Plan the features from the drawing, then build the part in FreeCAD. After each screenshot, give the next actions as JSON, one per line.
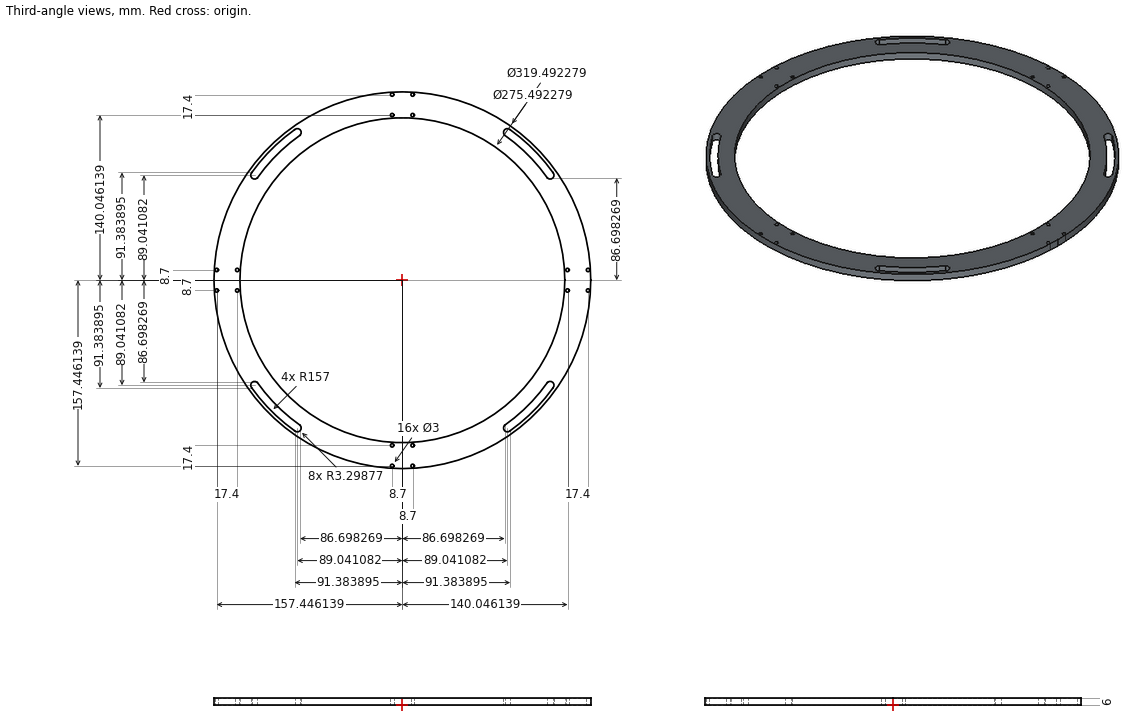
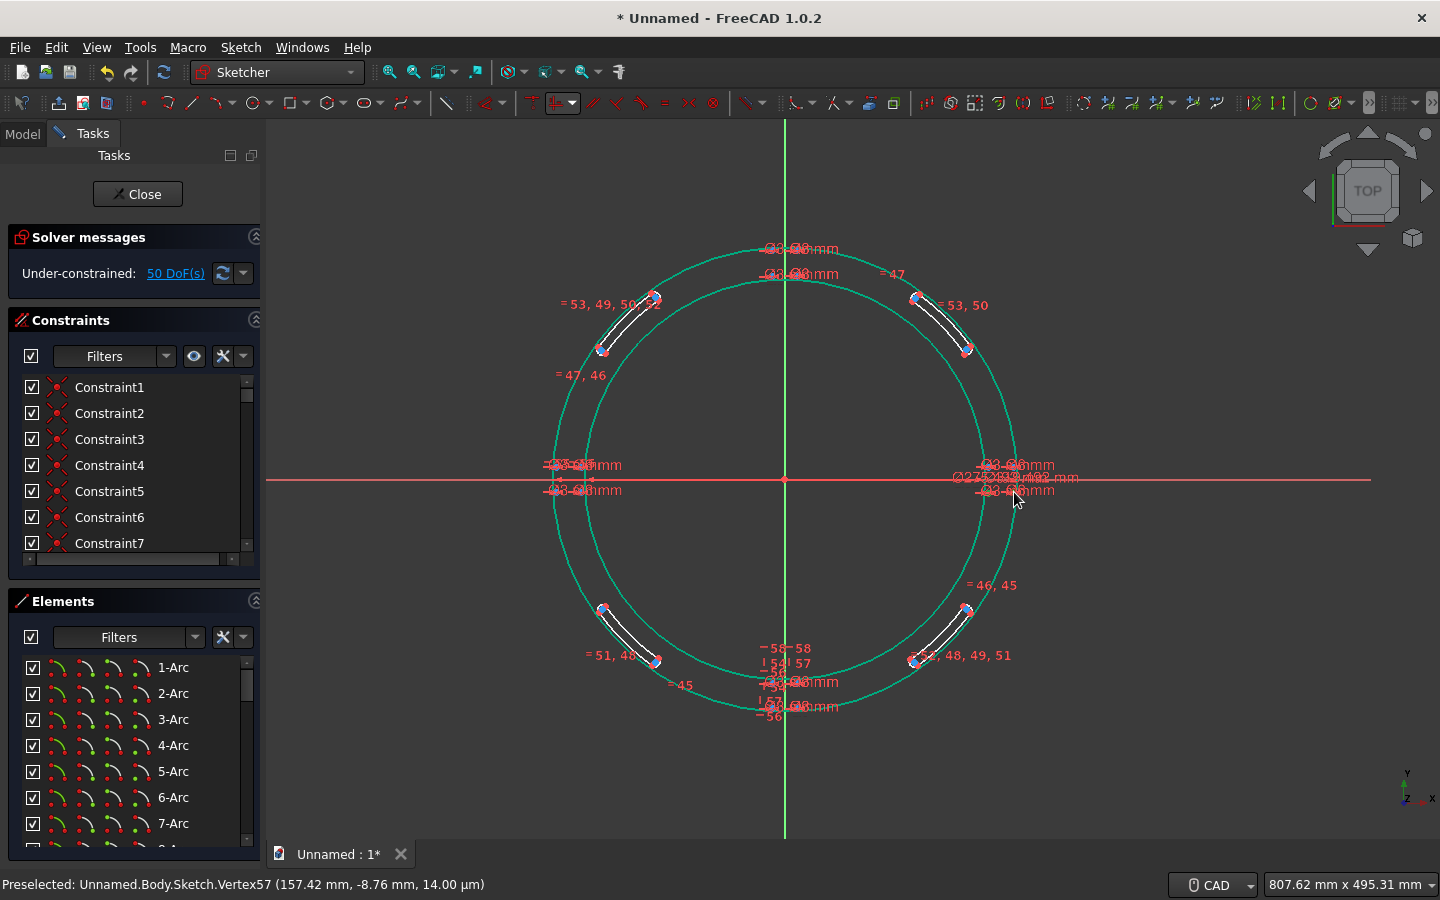
{"action": "left_click", "coordinate": [574, 104]}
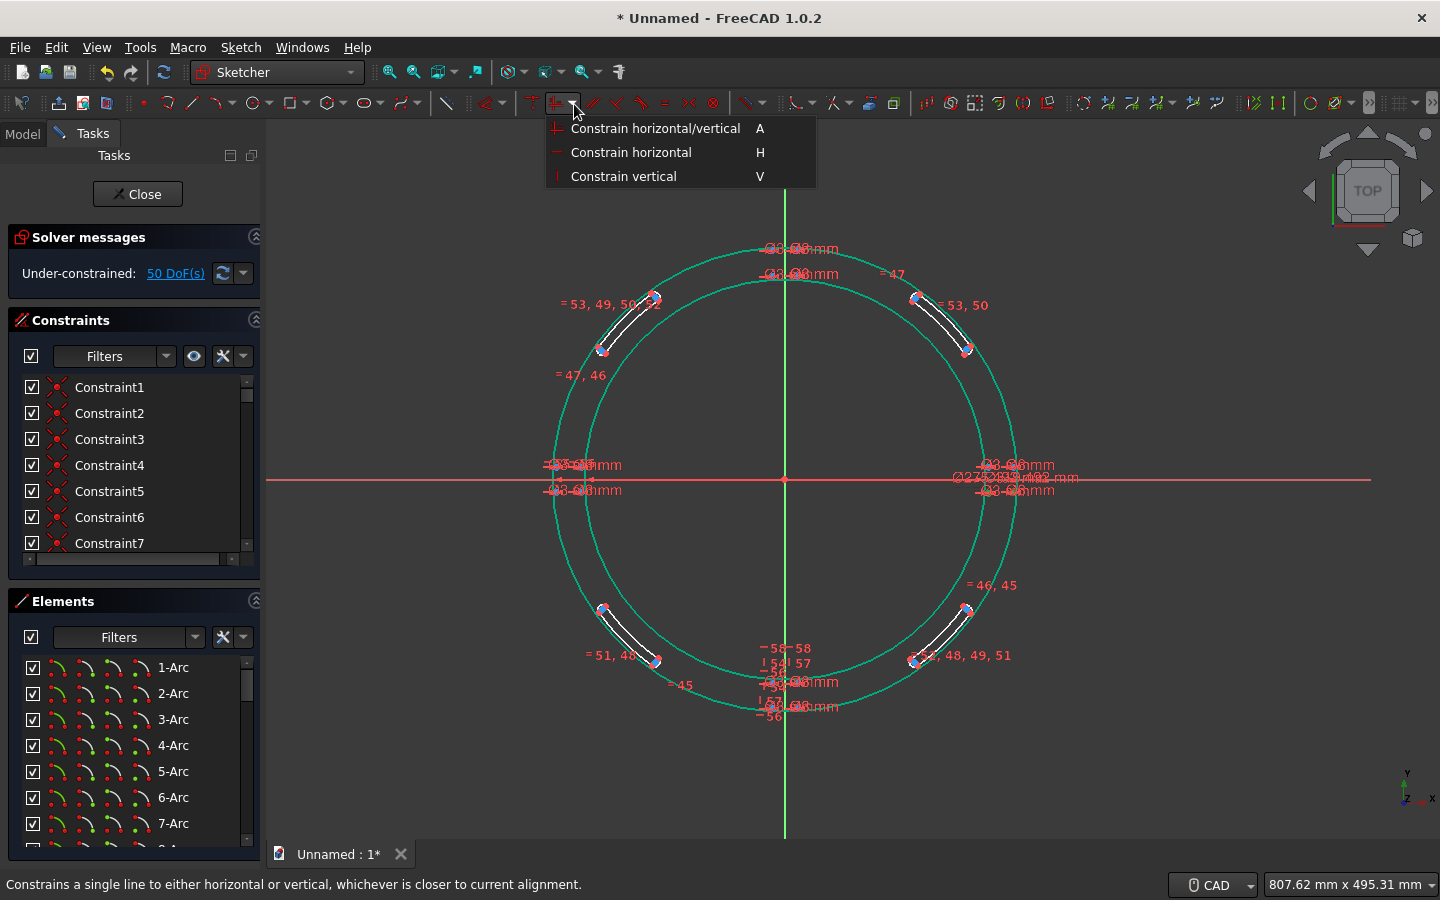
{"action": "left_click", "coordinate": [681, 152]}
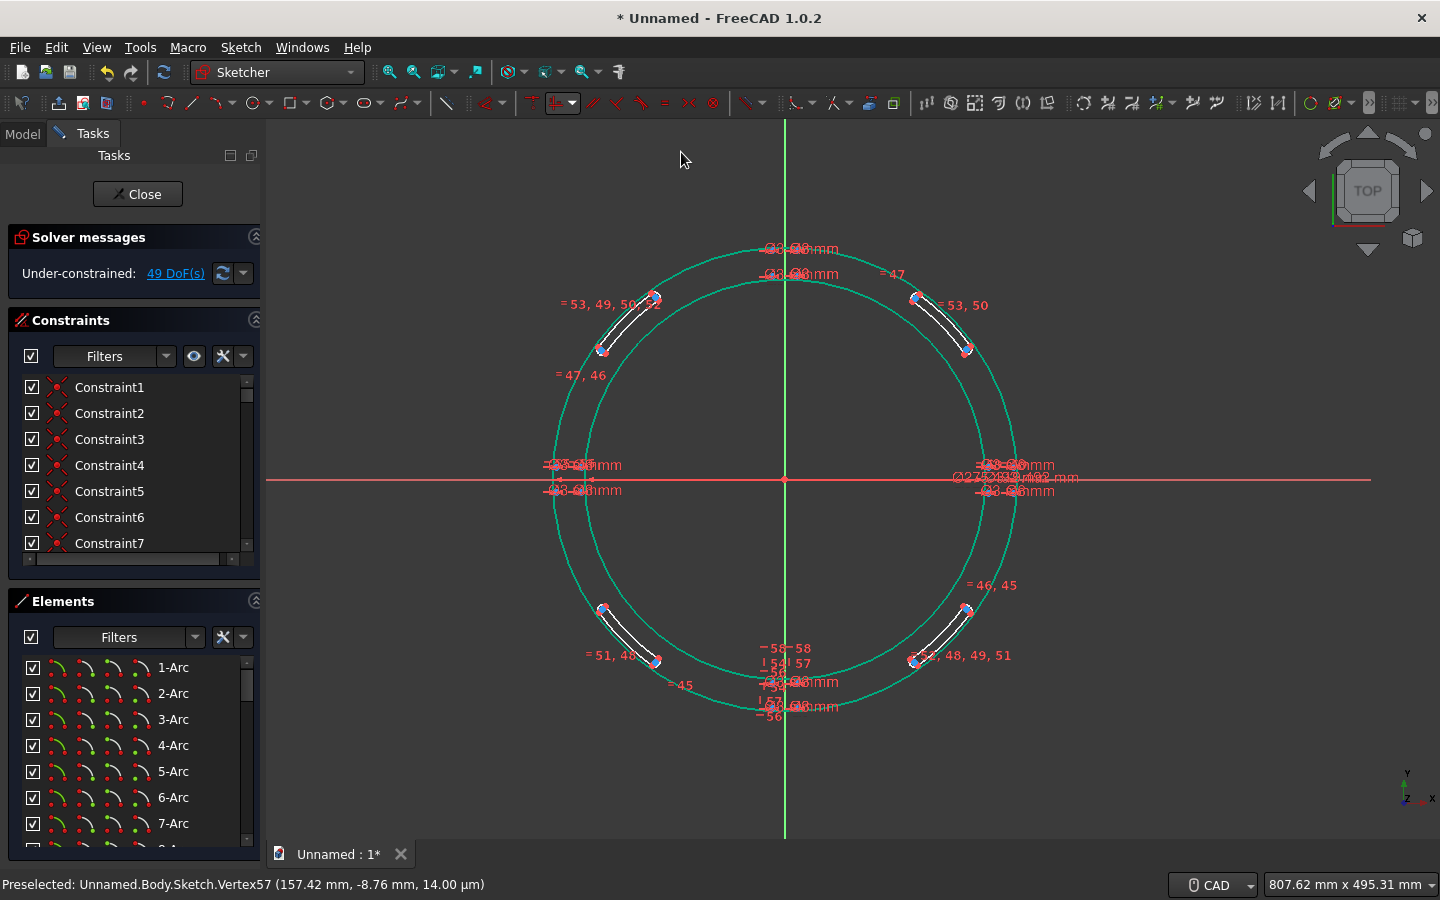
{"action": "left_click", "coordinate": [556, 492]}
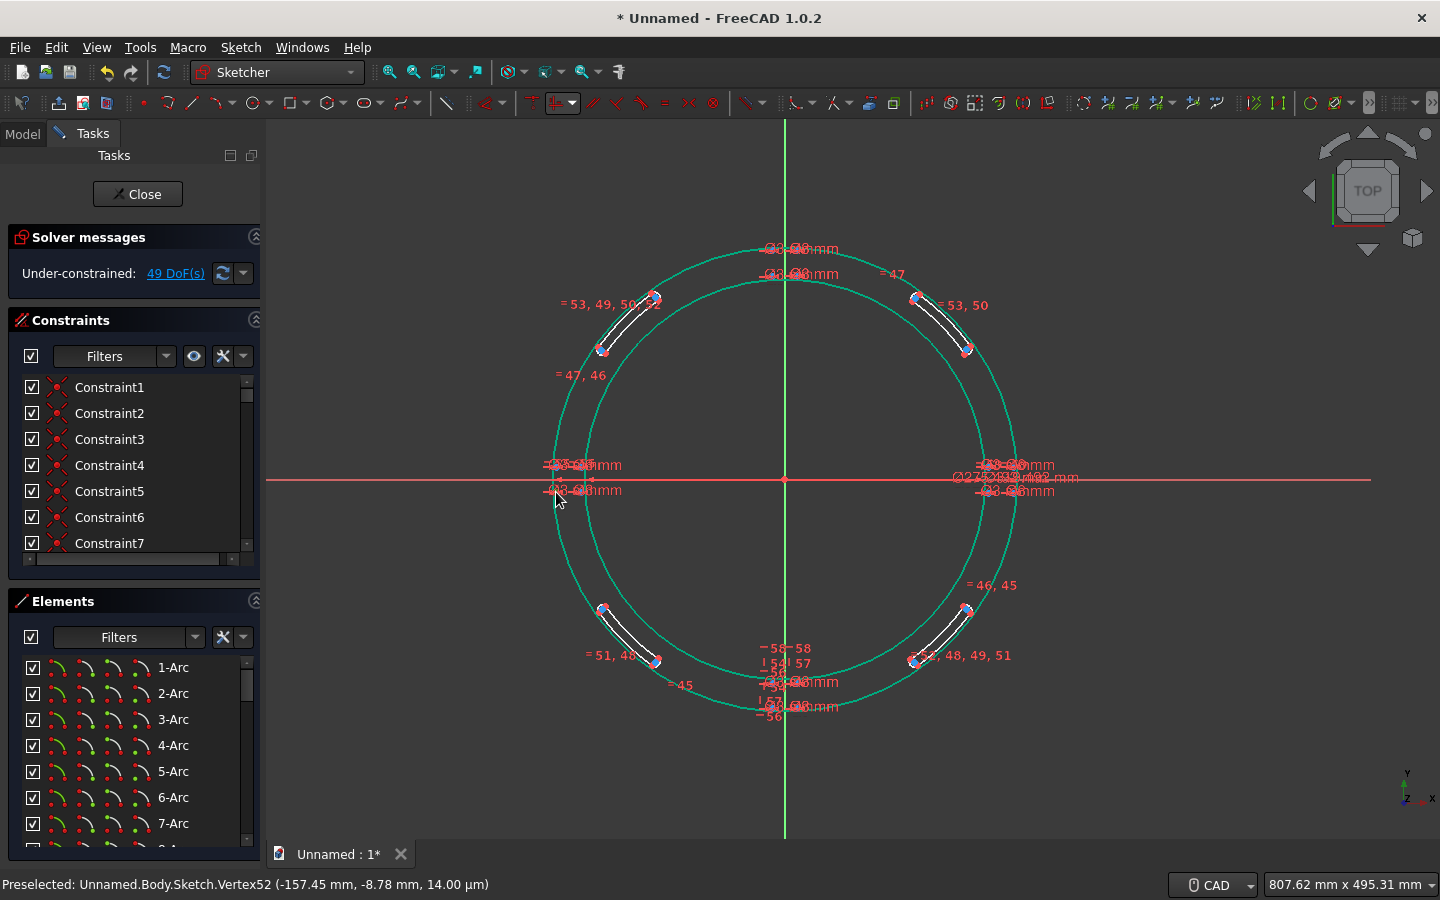
{"action": "left_click", "coordinate": [556, 467]}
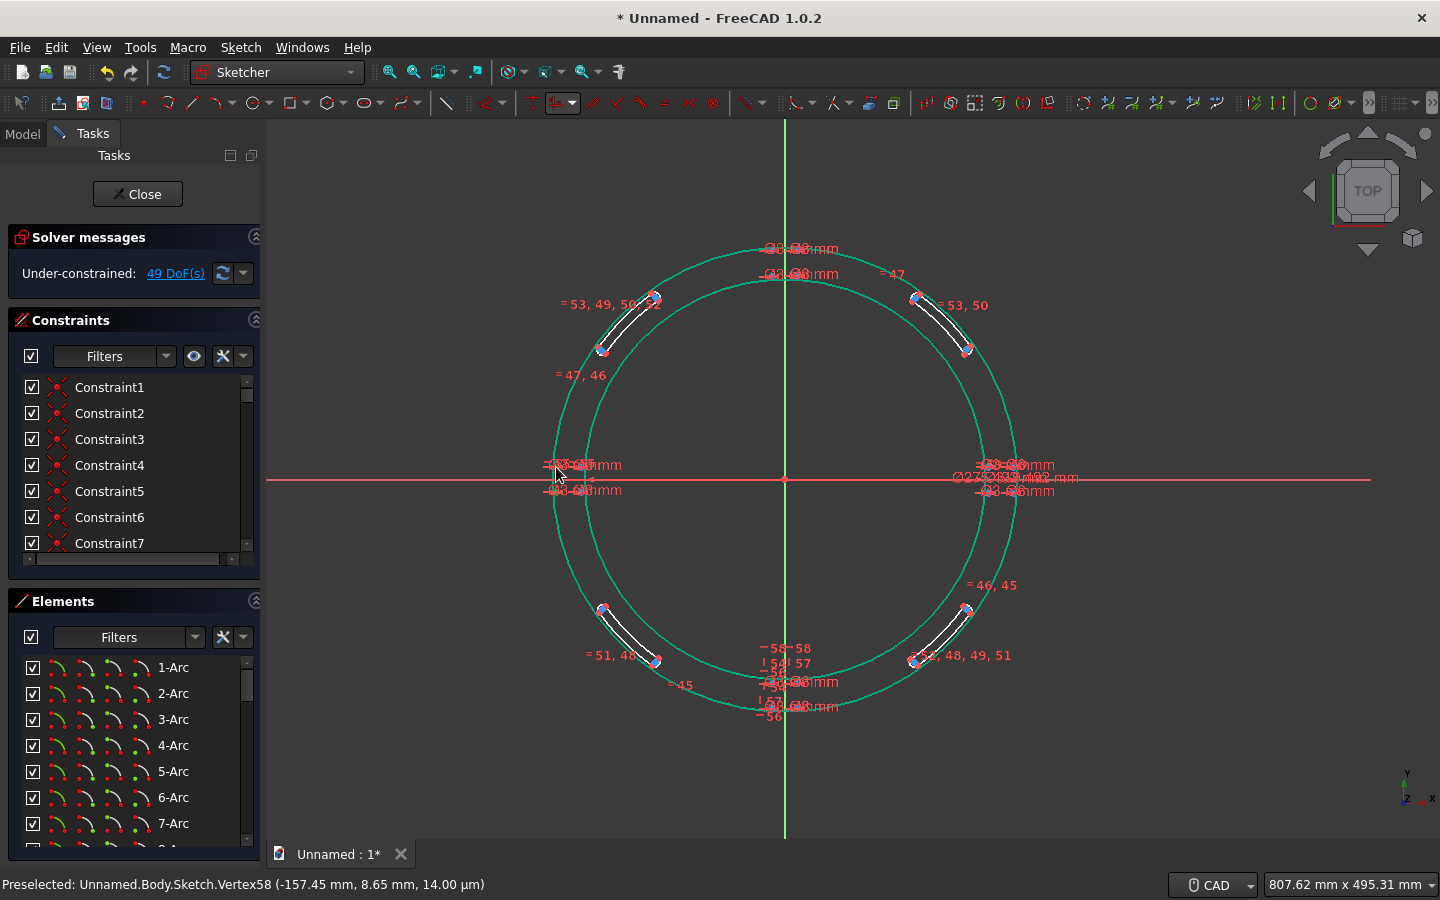
{"action": "key", "text": "v"}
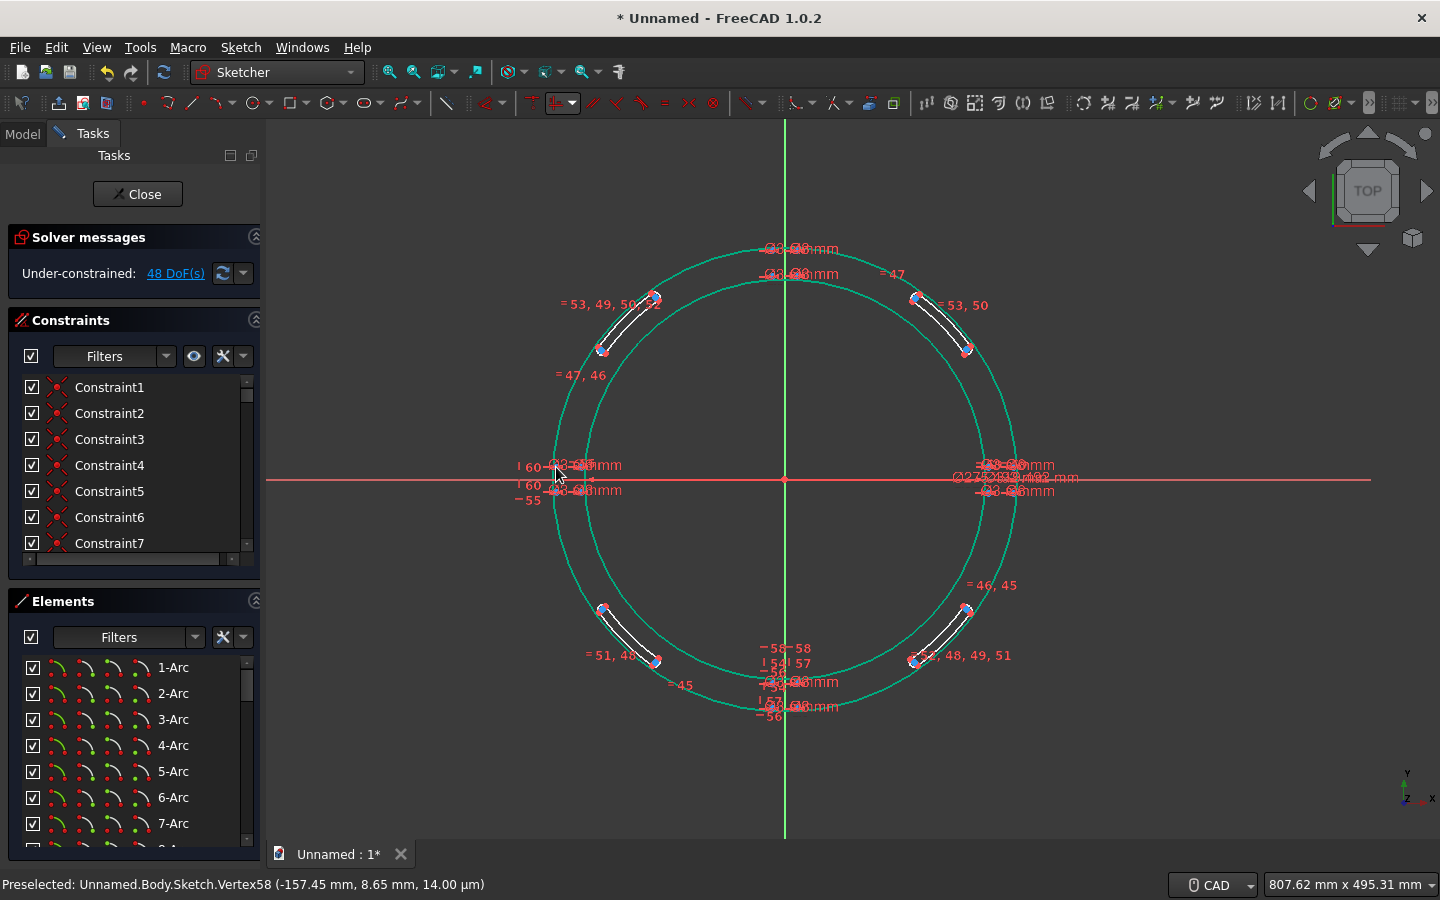
{"action": "left_click", "coordinate": [581, 492]}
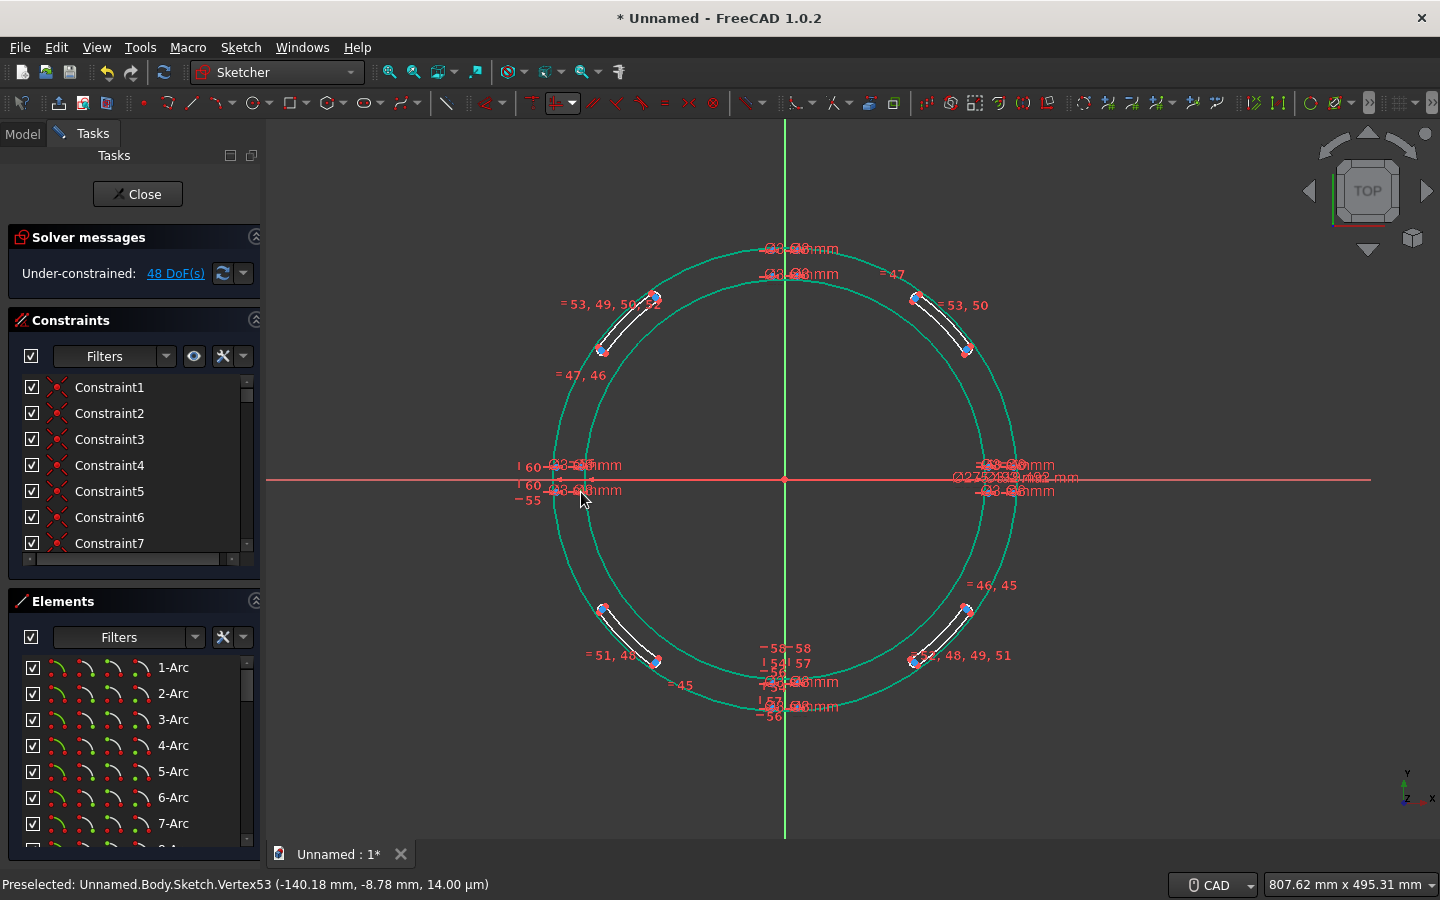
{"action": "scroll", "coordinate": [581, 467], "scroll_direction": "up", "scroll_amount": 4}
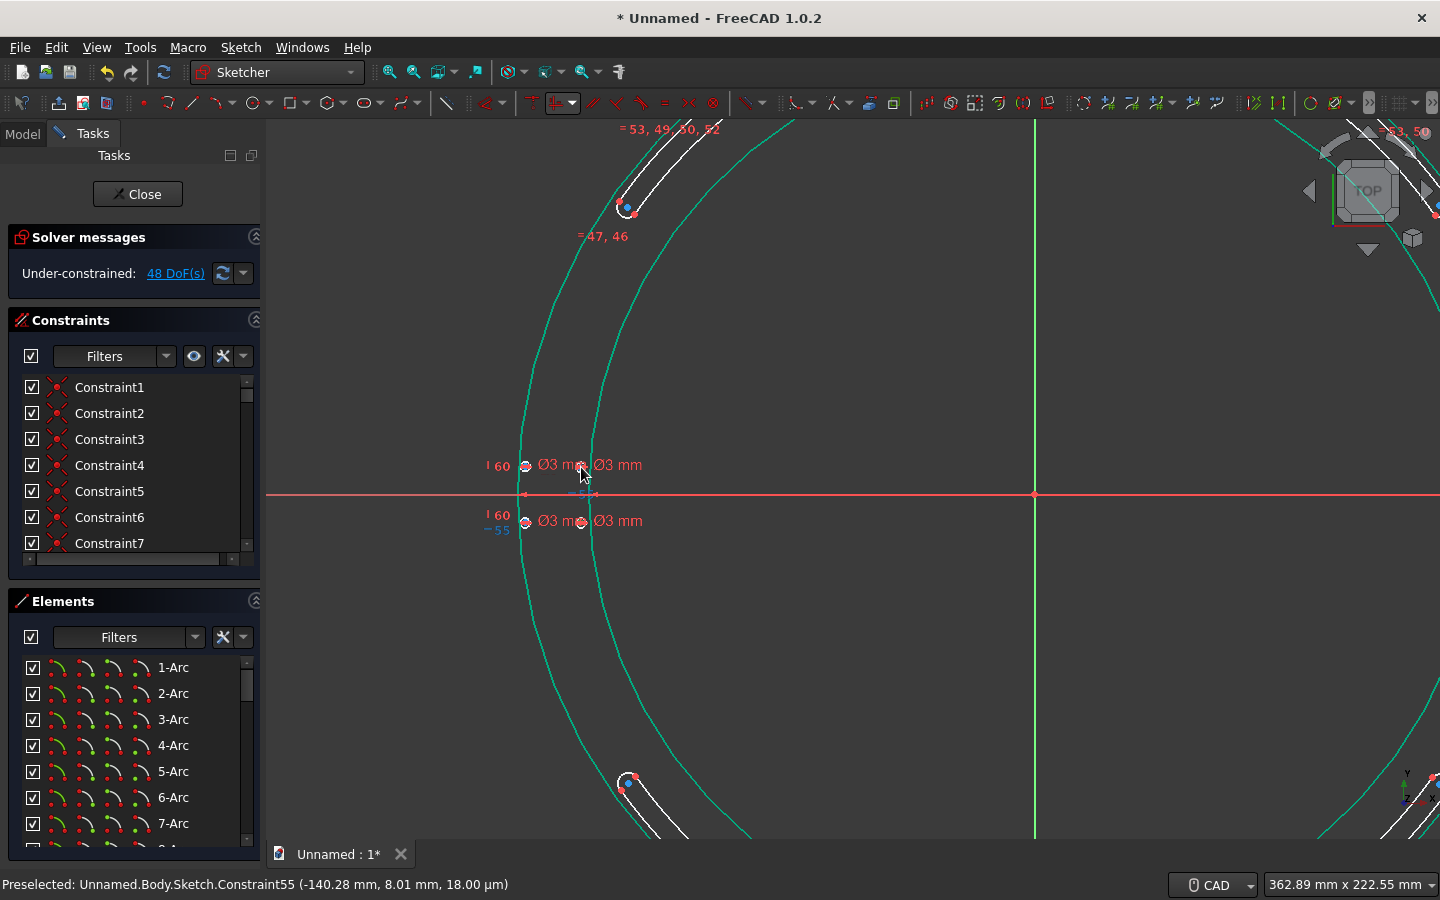
{"action": "left_click", "coordinate": [581, 467]}